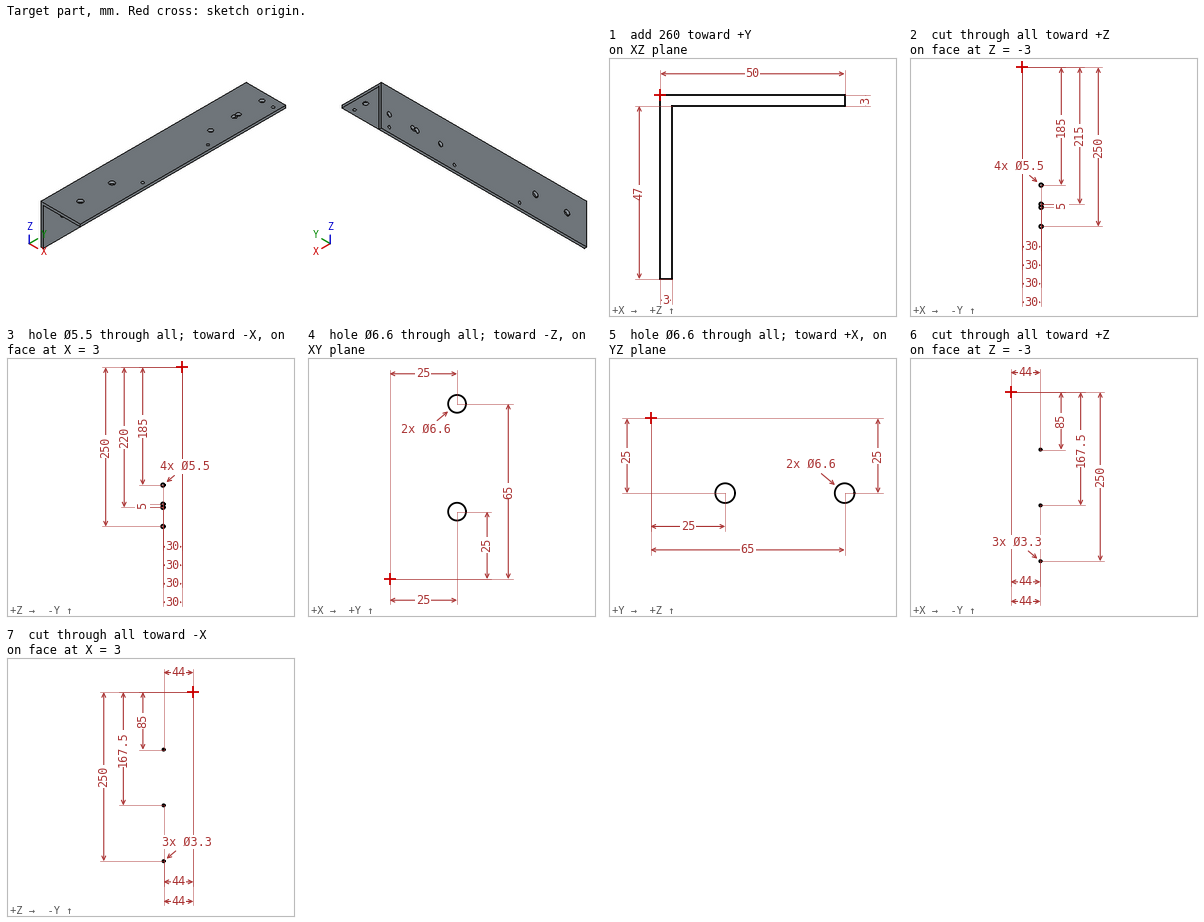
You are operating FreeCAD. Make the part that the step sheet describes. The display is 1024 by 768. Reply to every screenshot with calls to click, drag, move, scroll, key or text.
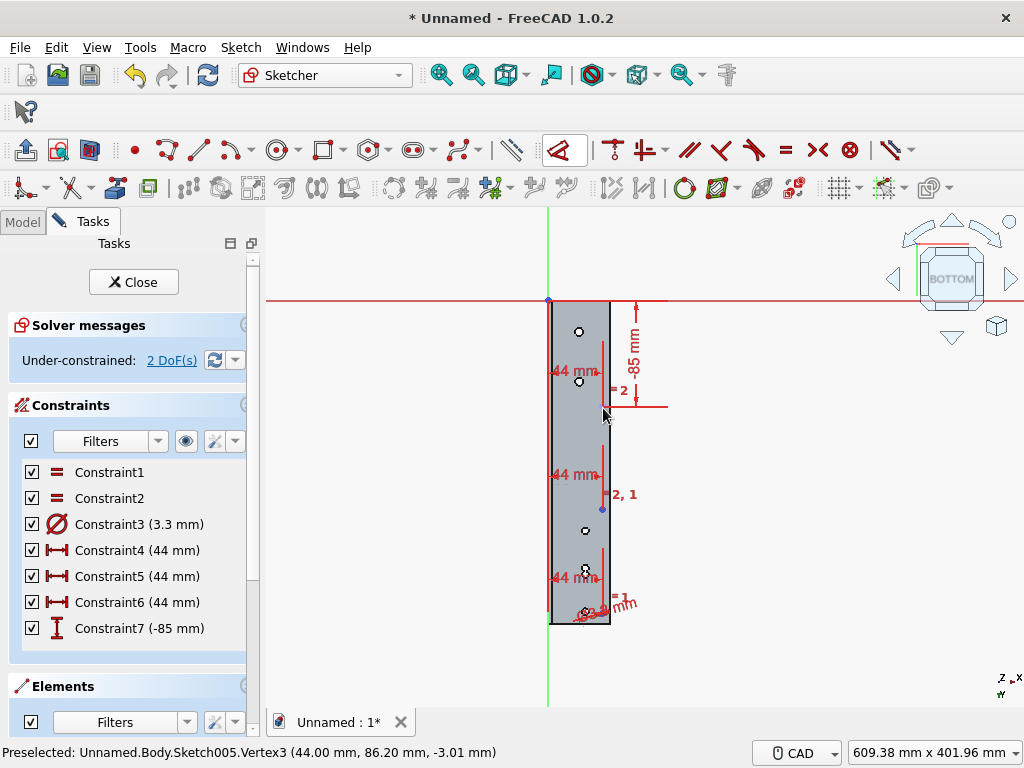
click(603, 613)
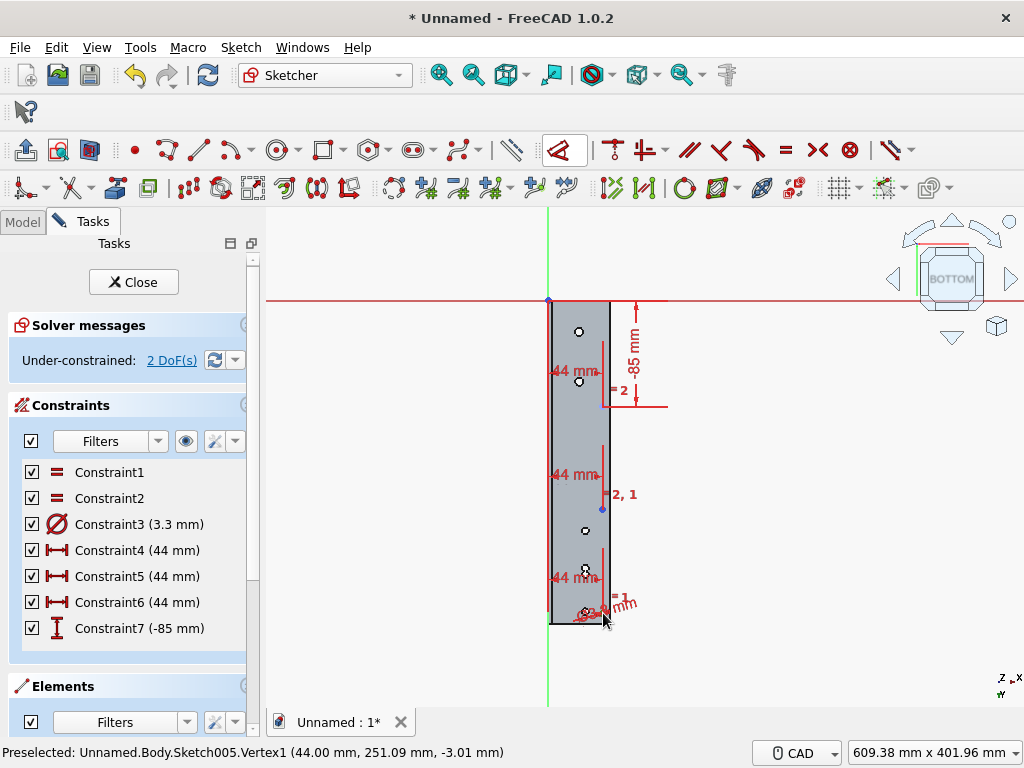
key(i)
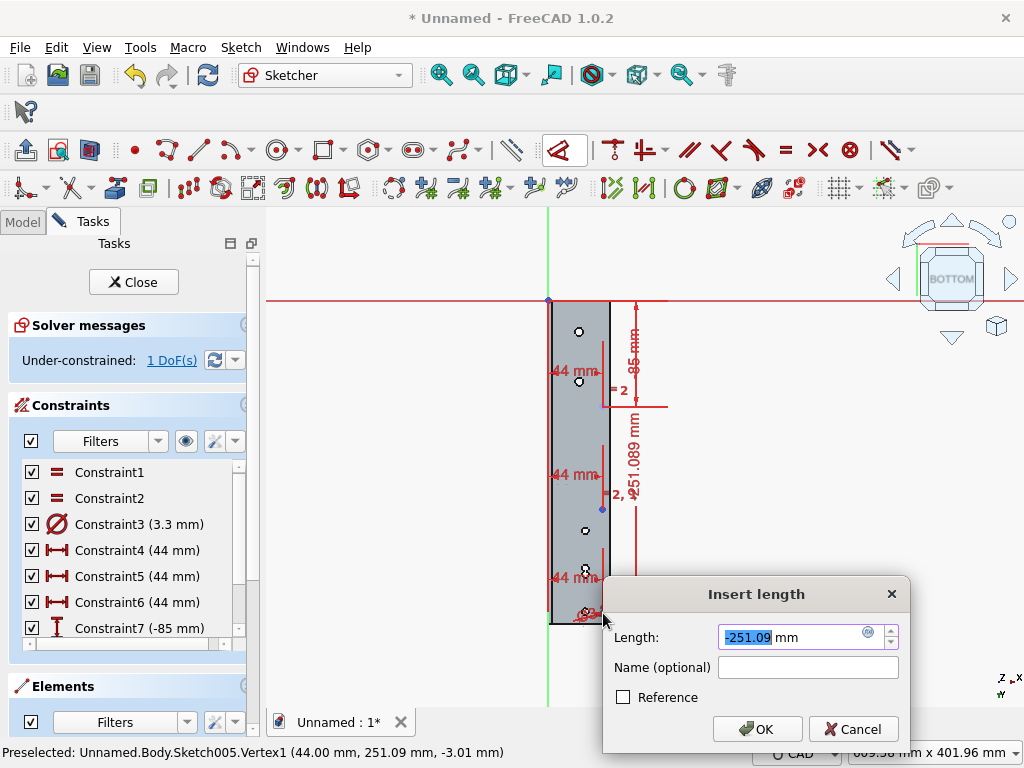
text(-250)
key(Return)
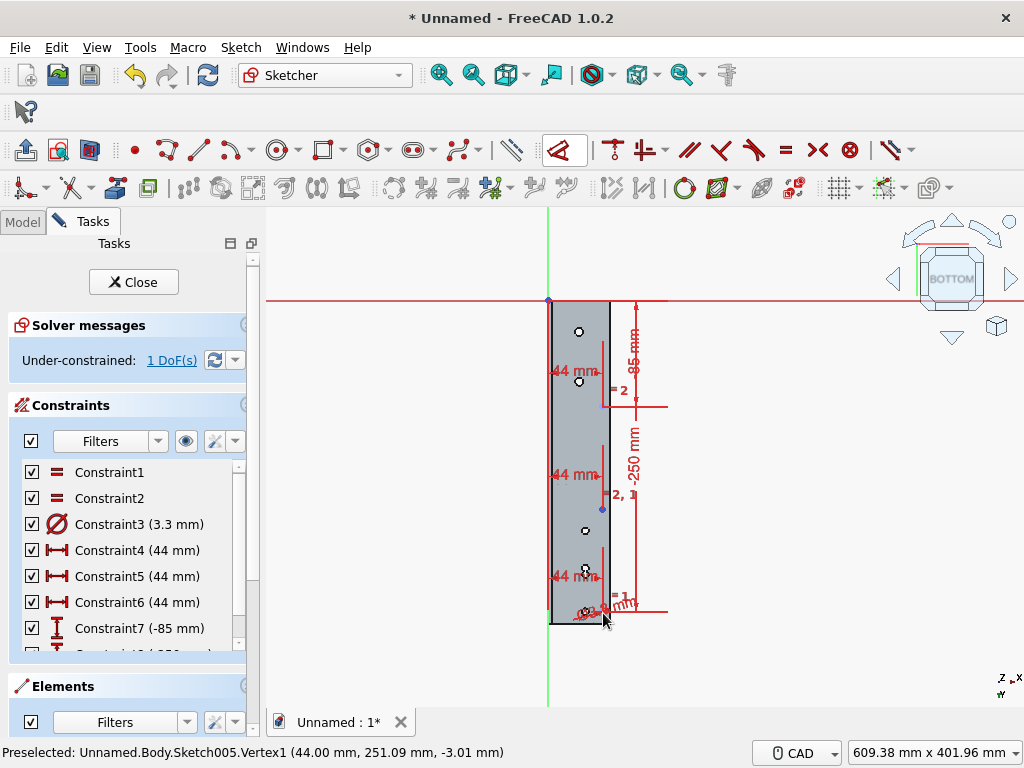
click(603, 510)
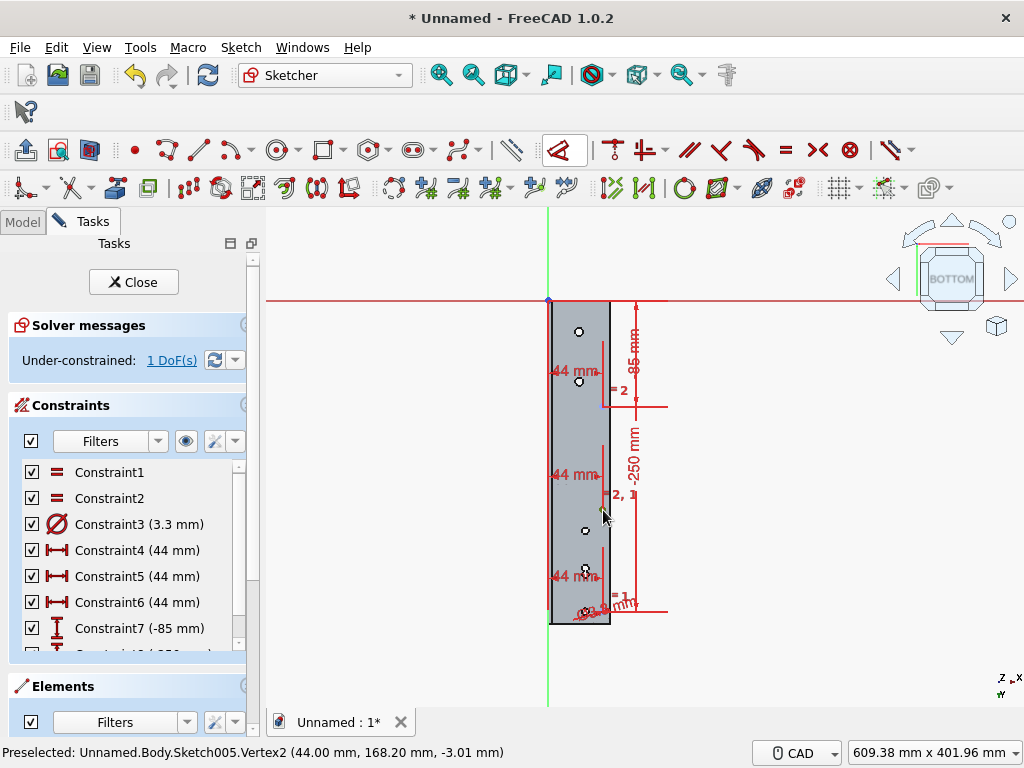
key(i)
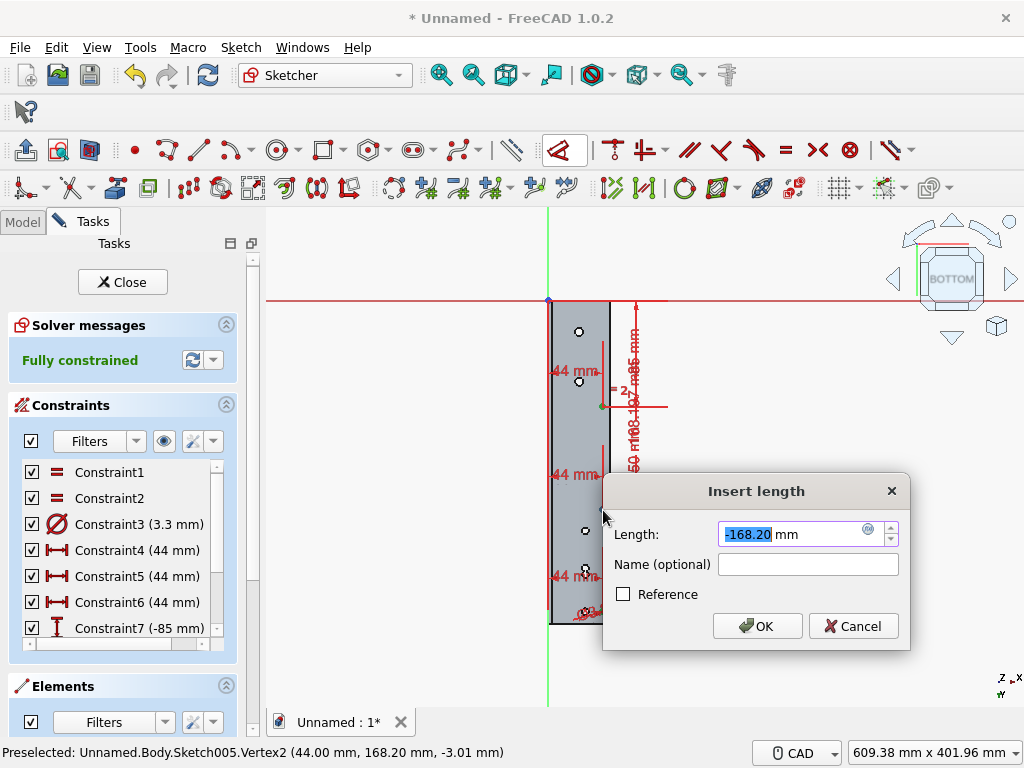
text(-167.5)
key(Return)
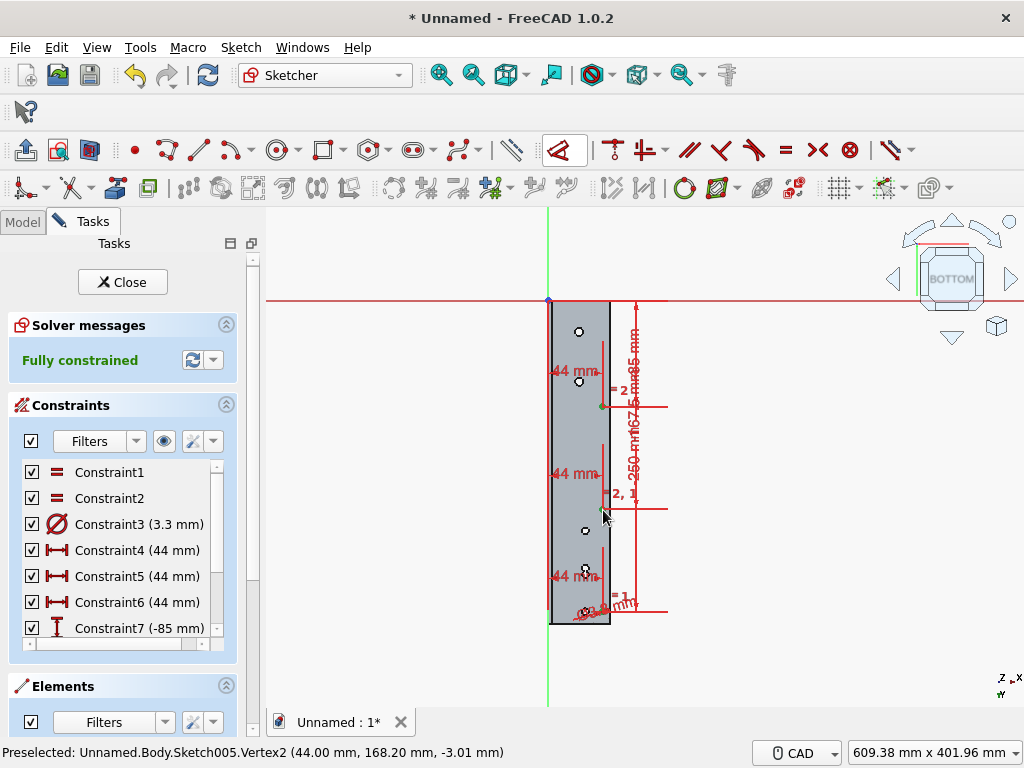
click(123, 282)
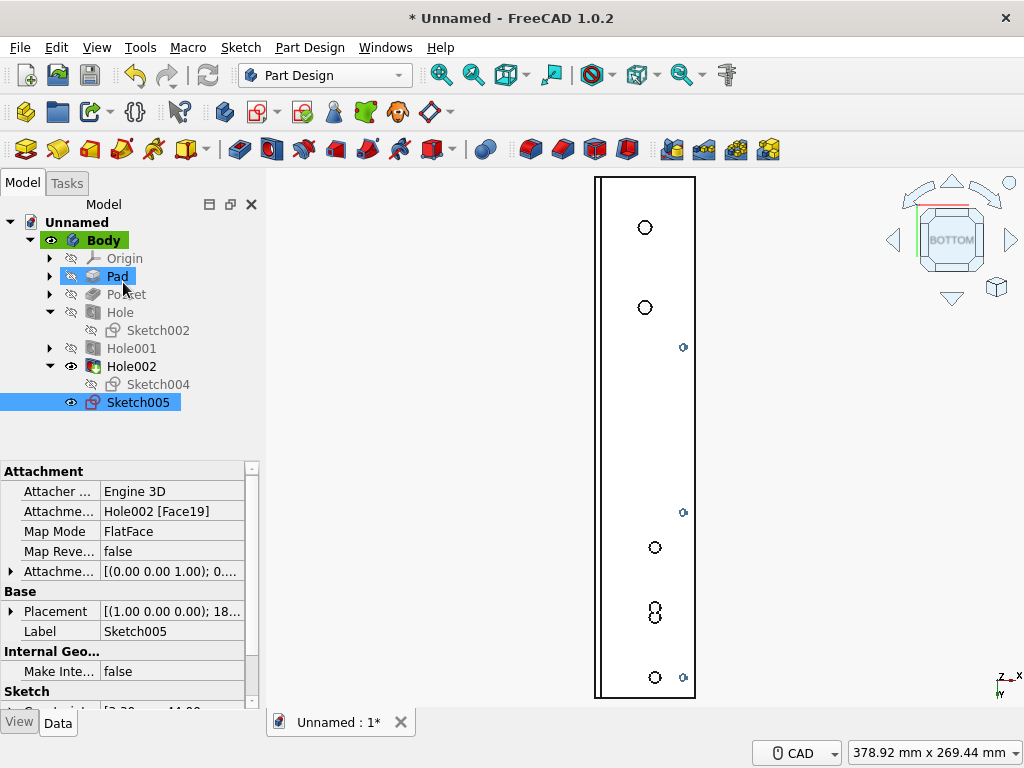
click(240, 150)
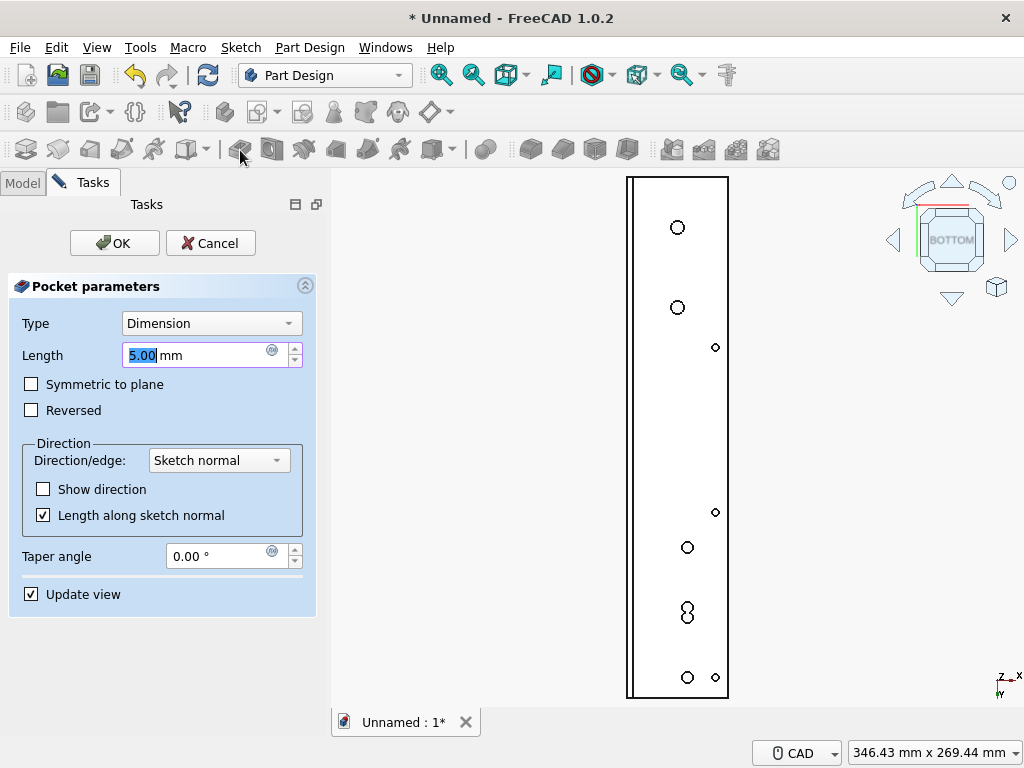
click(212, 324)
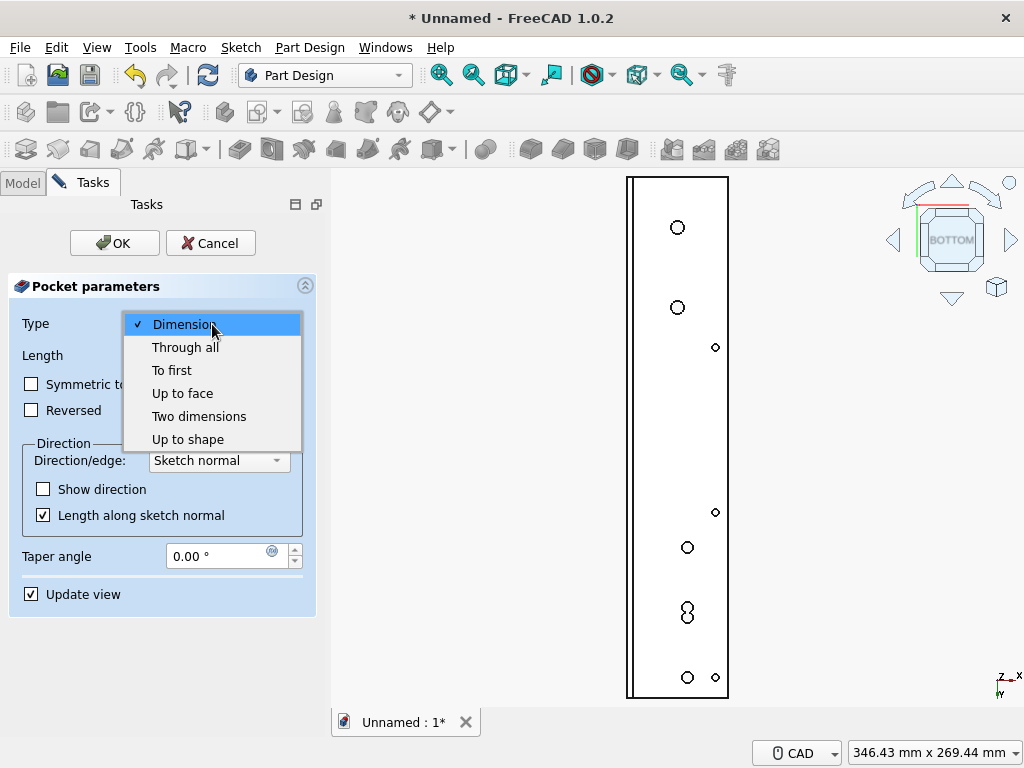
click(212, 348)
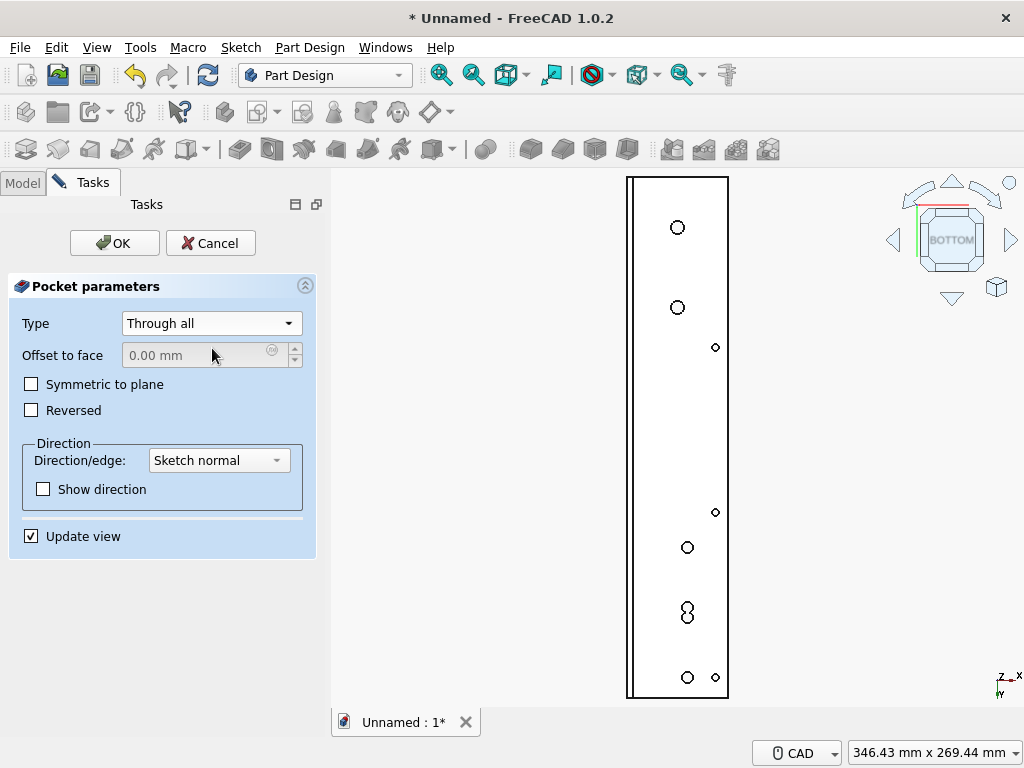
click(115, 243)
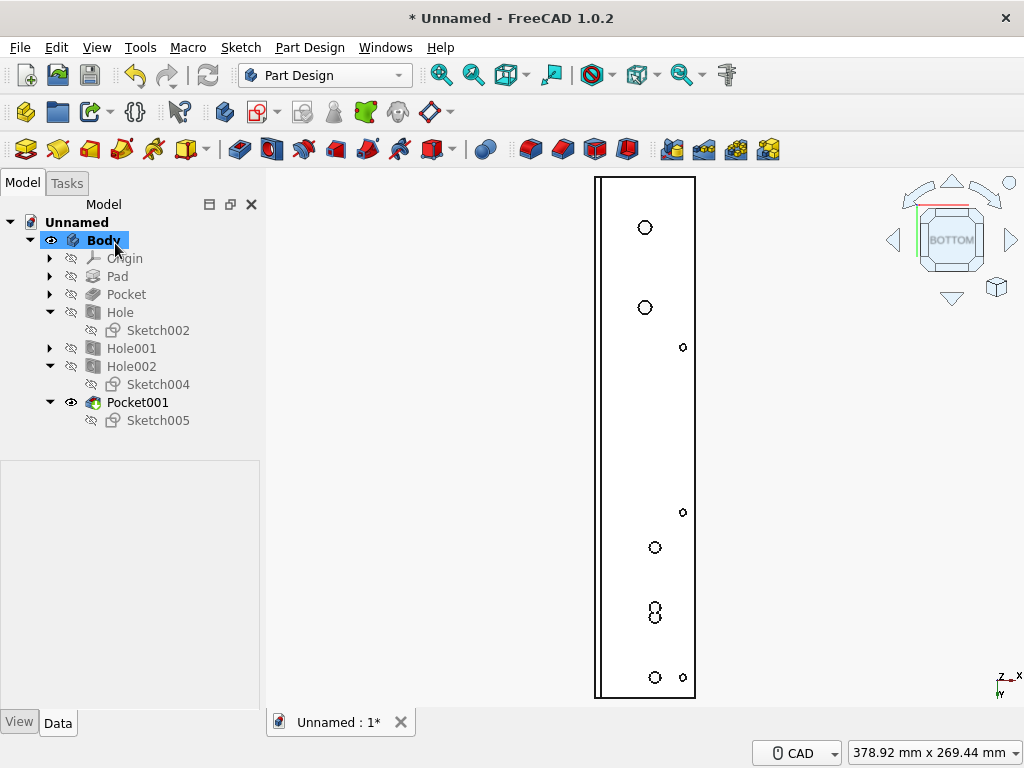
key(0)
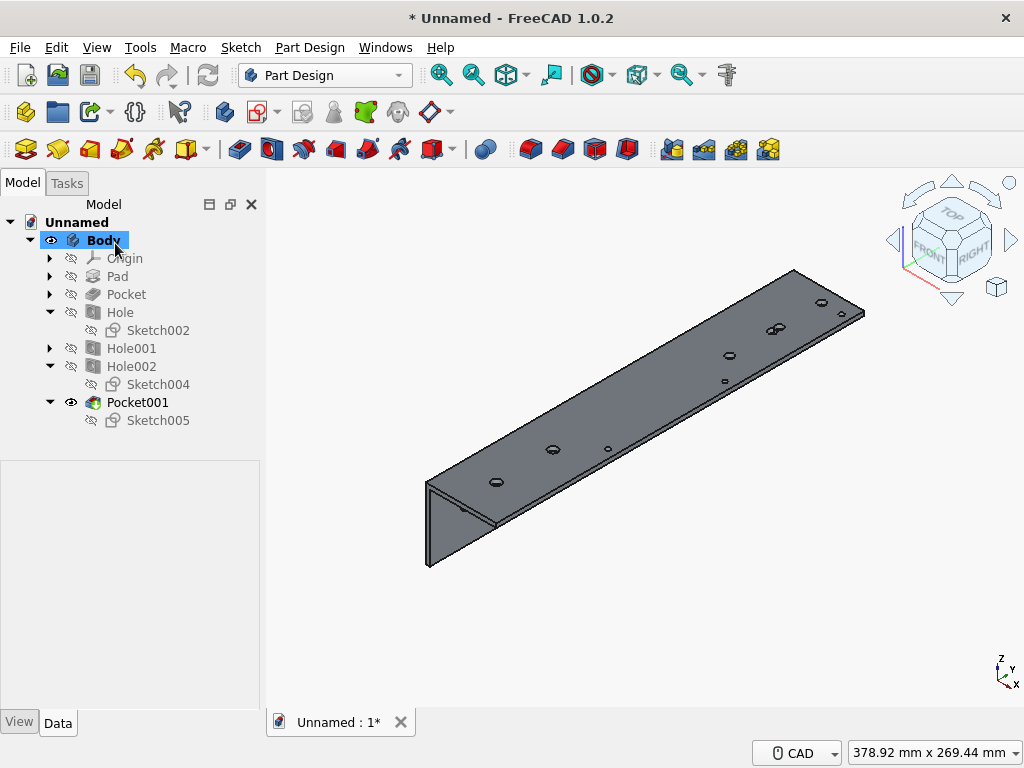
key(3)